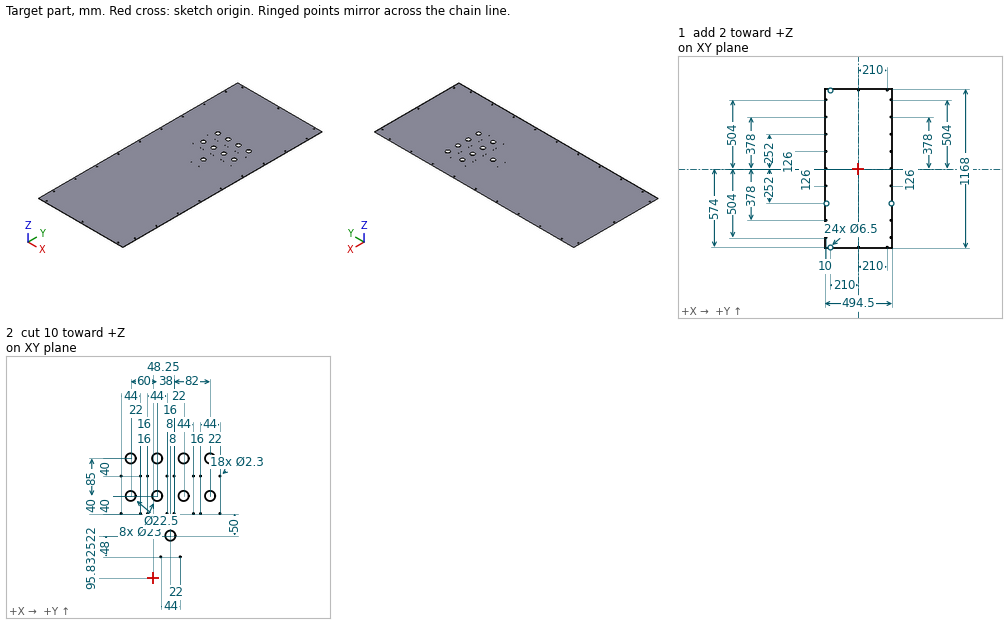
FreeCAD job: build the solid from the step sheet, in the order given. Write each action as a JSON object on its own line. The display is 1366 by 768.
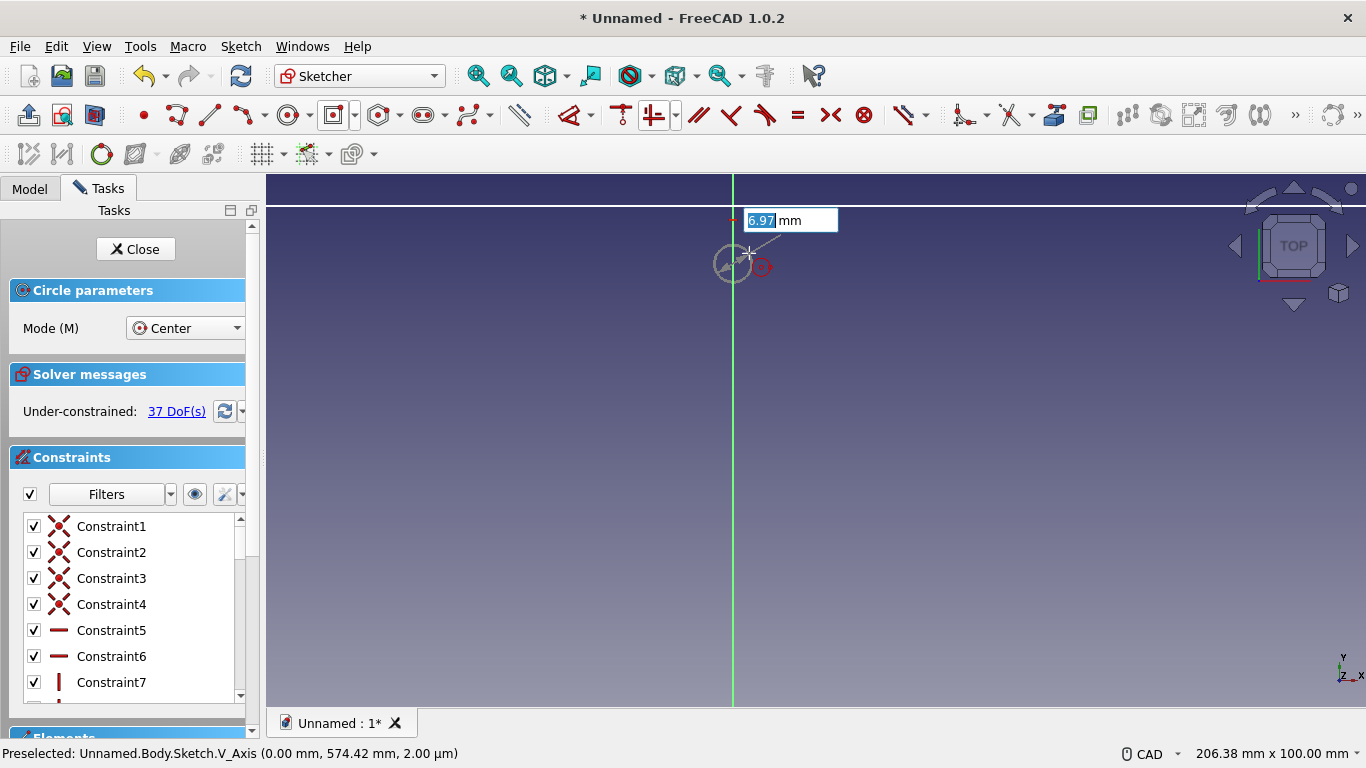
{"action": "type", "text": "6.5"}
{"action": "key", "text": "Return"}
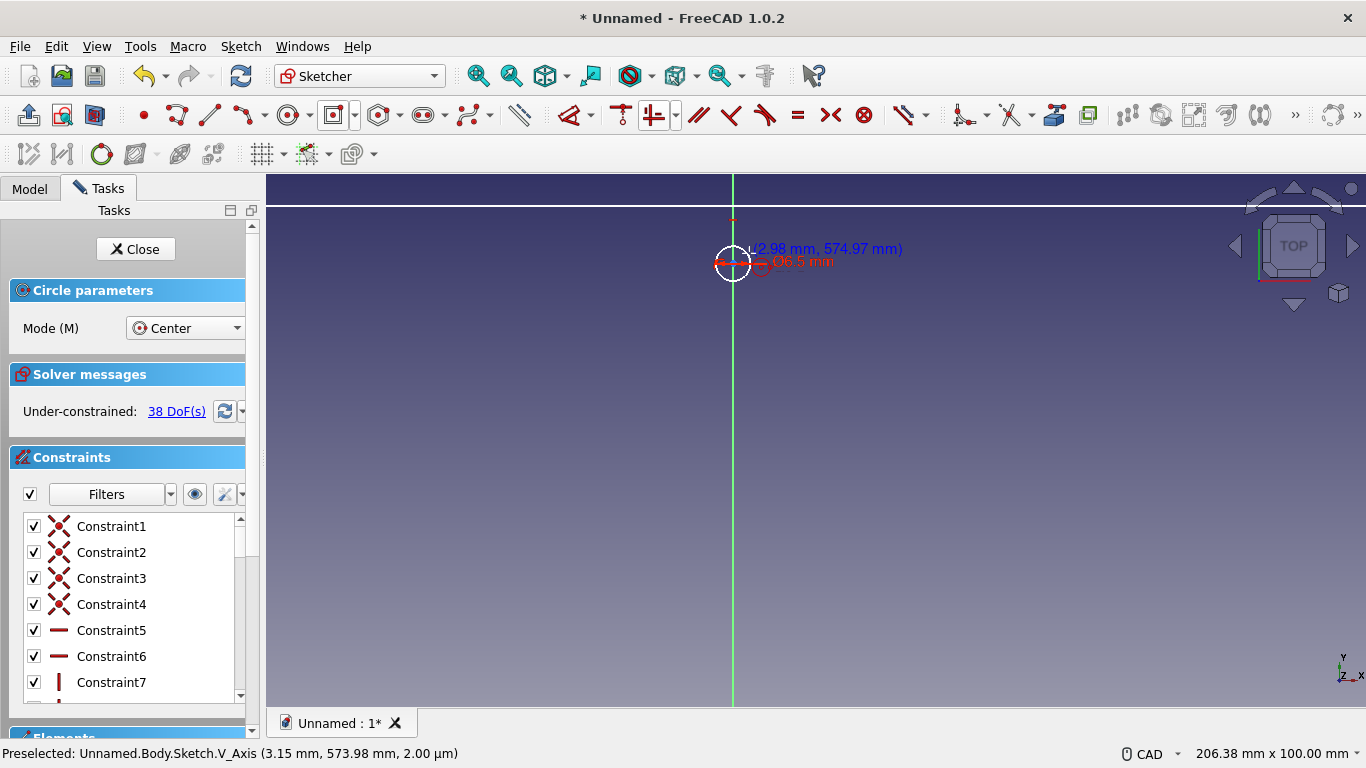
{"action": "scroll", "coordinate": [748, 290], "scroll_direction": "down", "scroll_amount": 15}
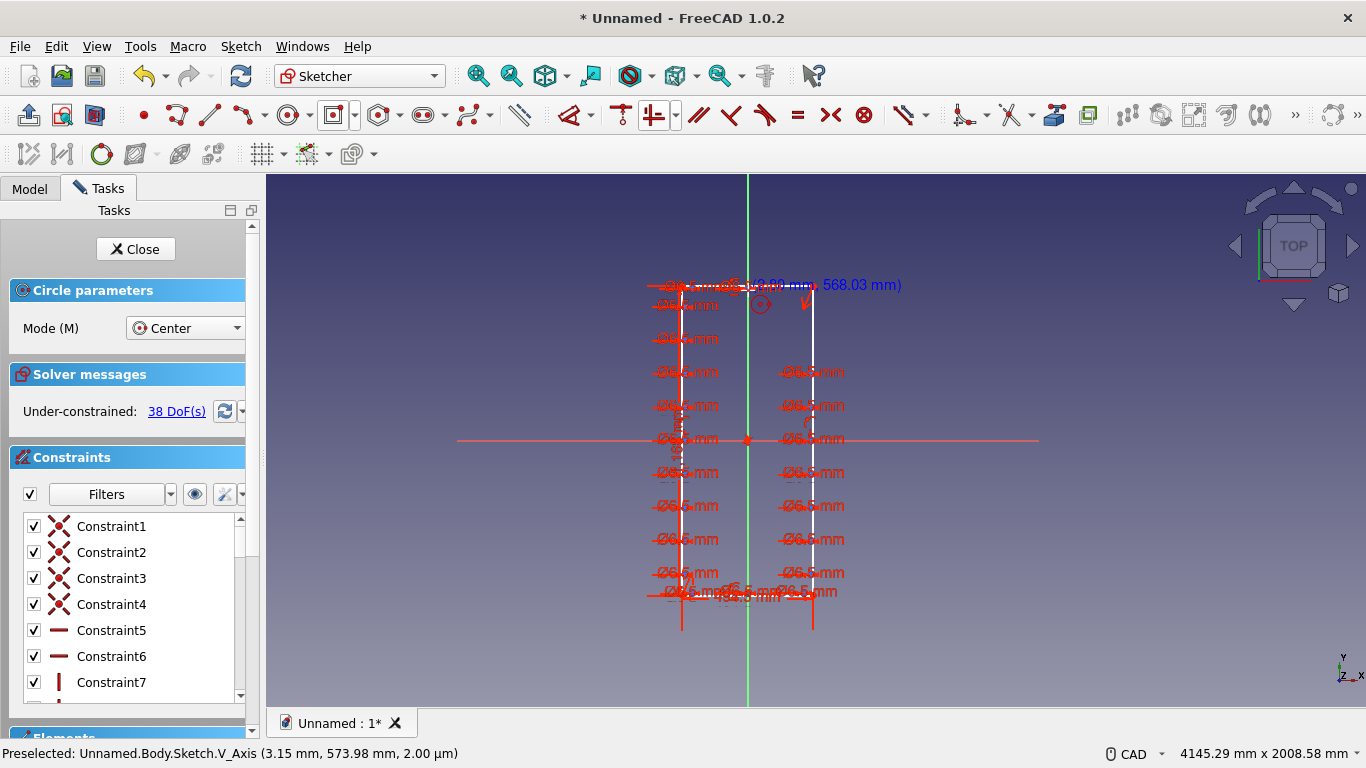
{"action": "scroll", "coordinate": [811, 341], "scroll_direction": "up", "scroll_amount": 17}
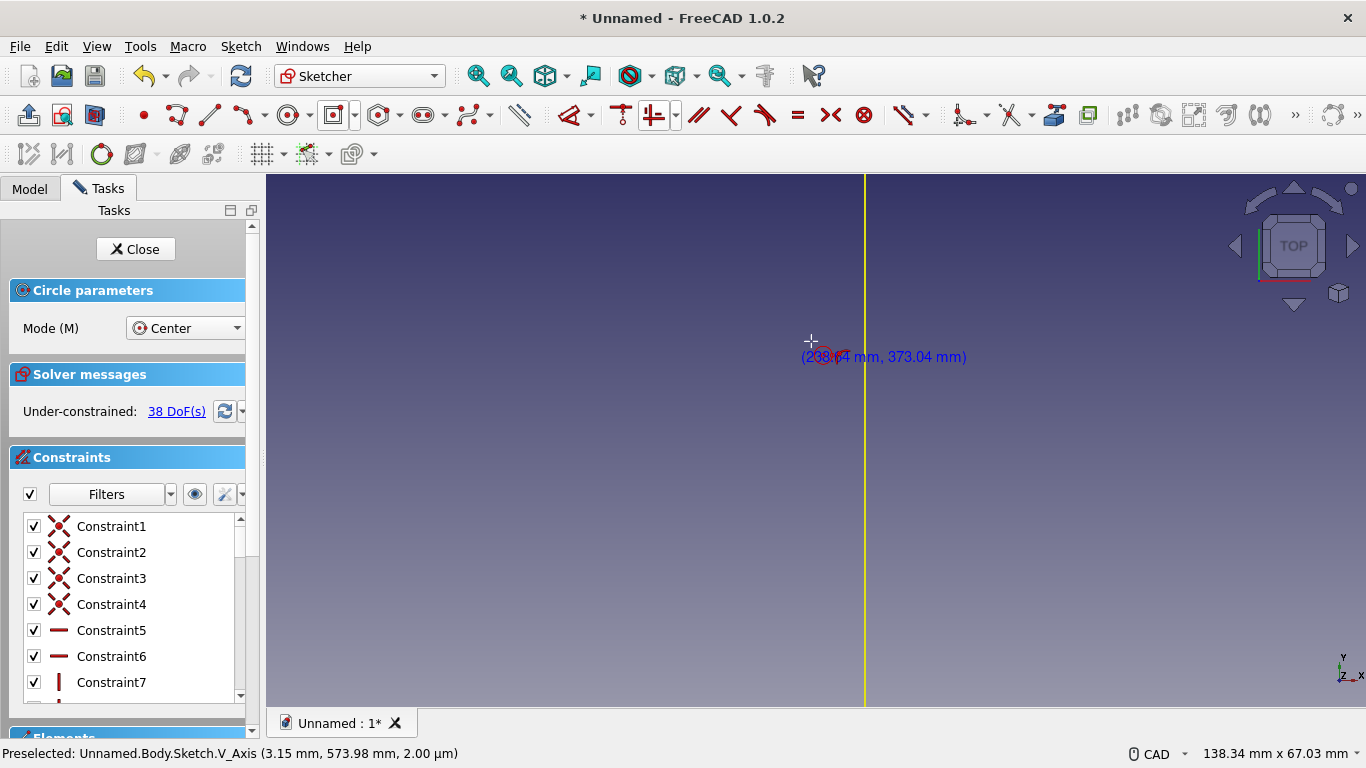
{"action": "scroll", "coordinate": [826, 318], "scroll_direction": "down", "scroll_amount": 16}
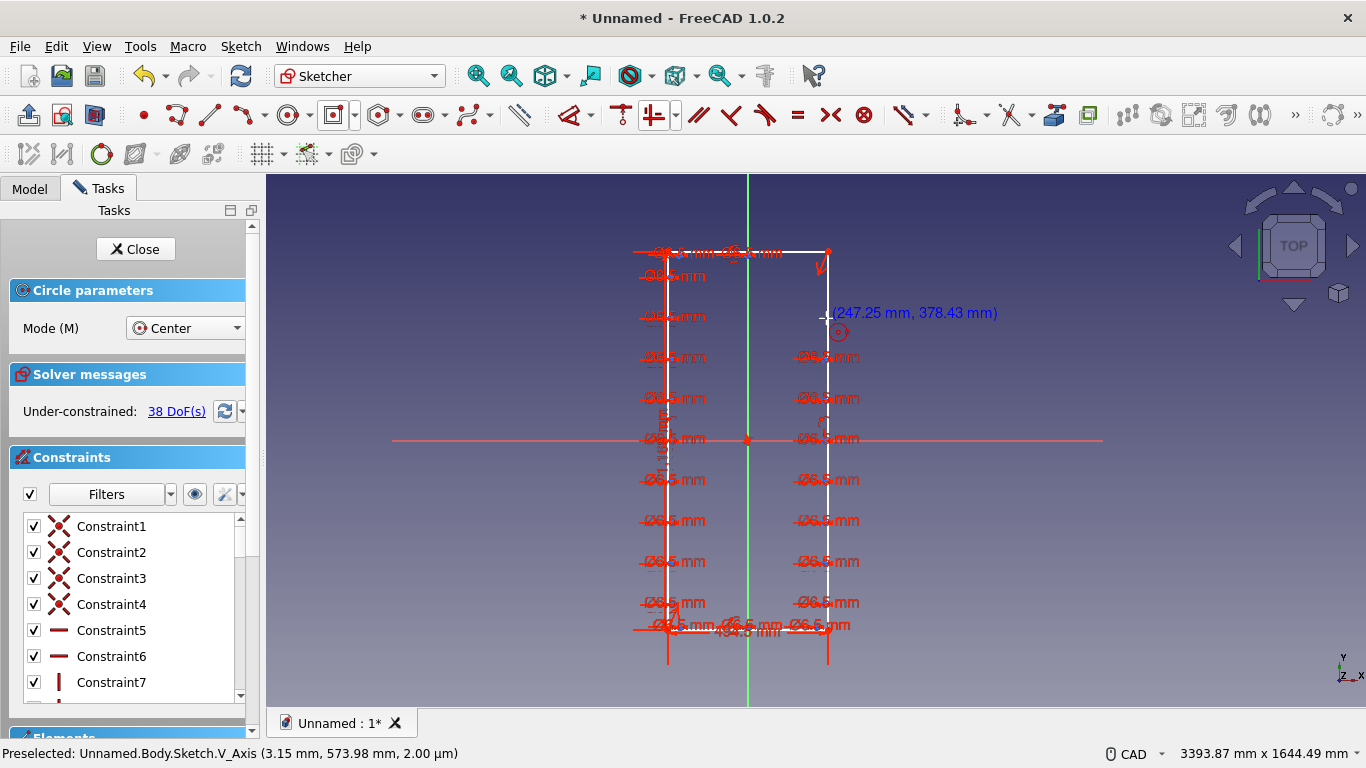
{"action": "scroll", "coordinate": [825, 318], "scroll_direction": "up", "scroll_amount": 8}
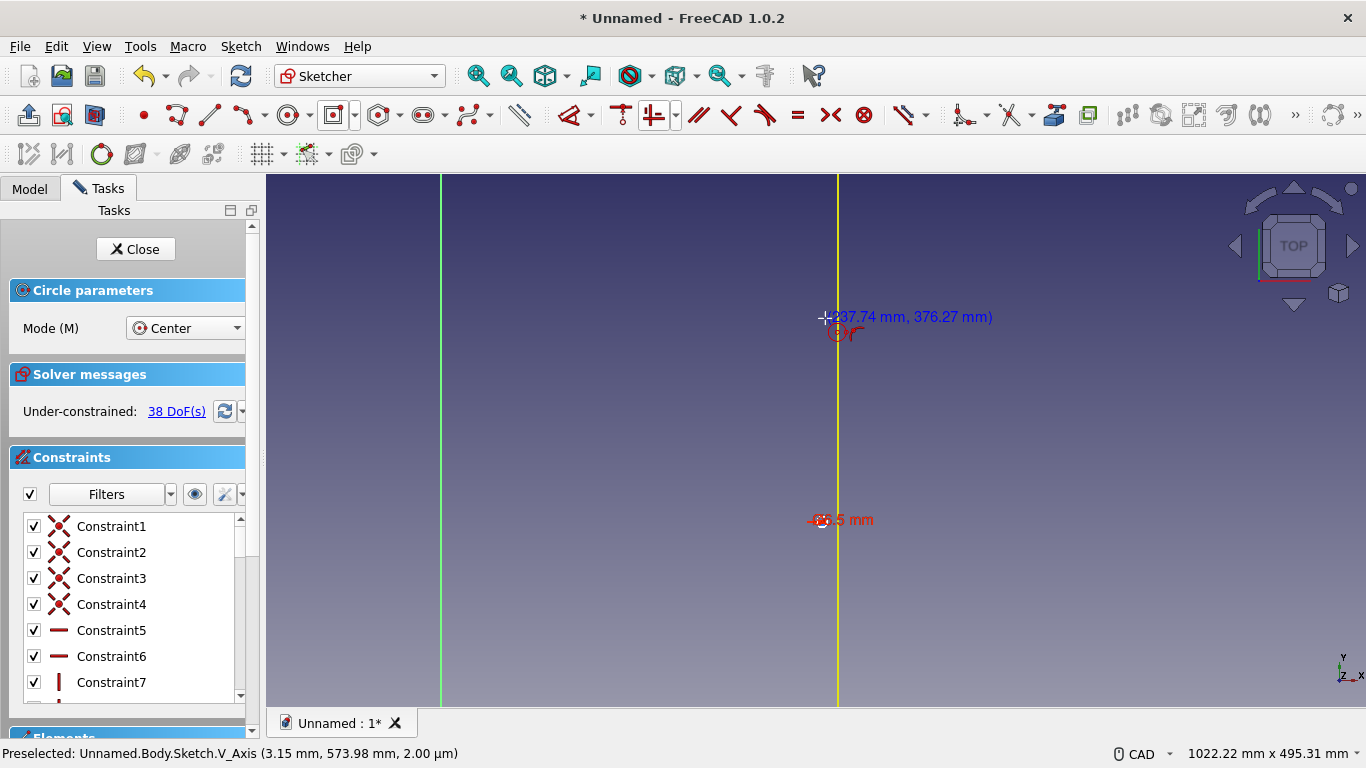
{"action": "left_click", "coordinate": [822, 319]}
{"action": "mouse_move", "coordinate": [819, 315]}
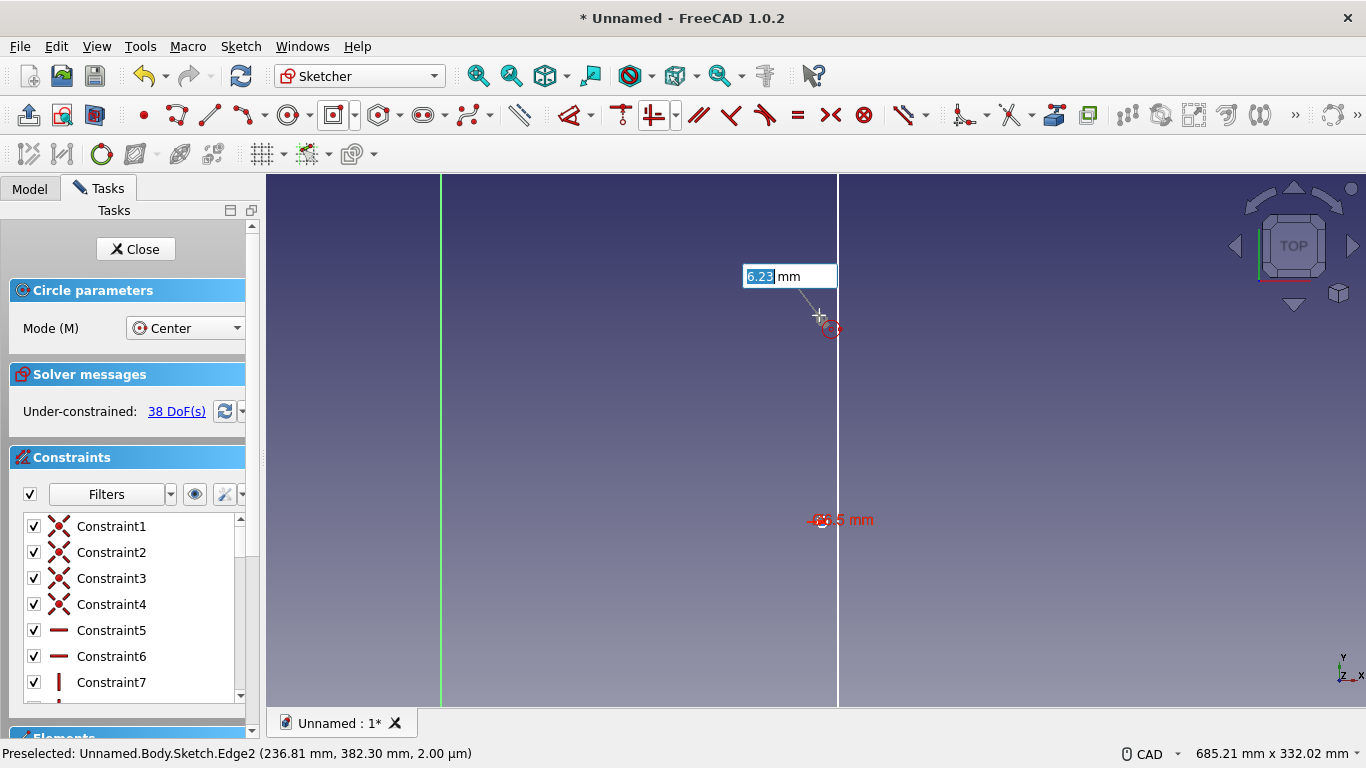
{"action": "type", "text": "6.5"}
{"action": "key", "text": "Return"}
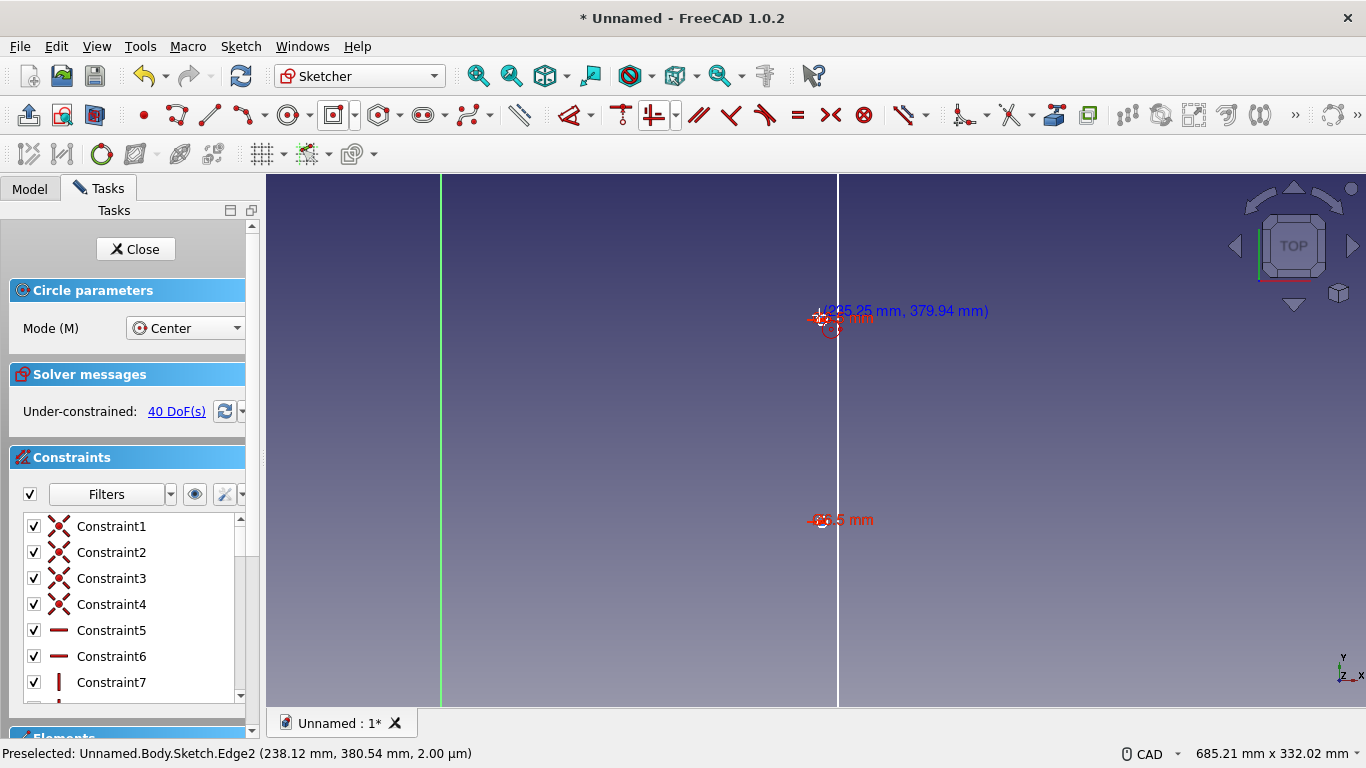
{"action": "scroll", "coordinate": [808, 344], "scroll_direction": "down", "scroll_amount": 9}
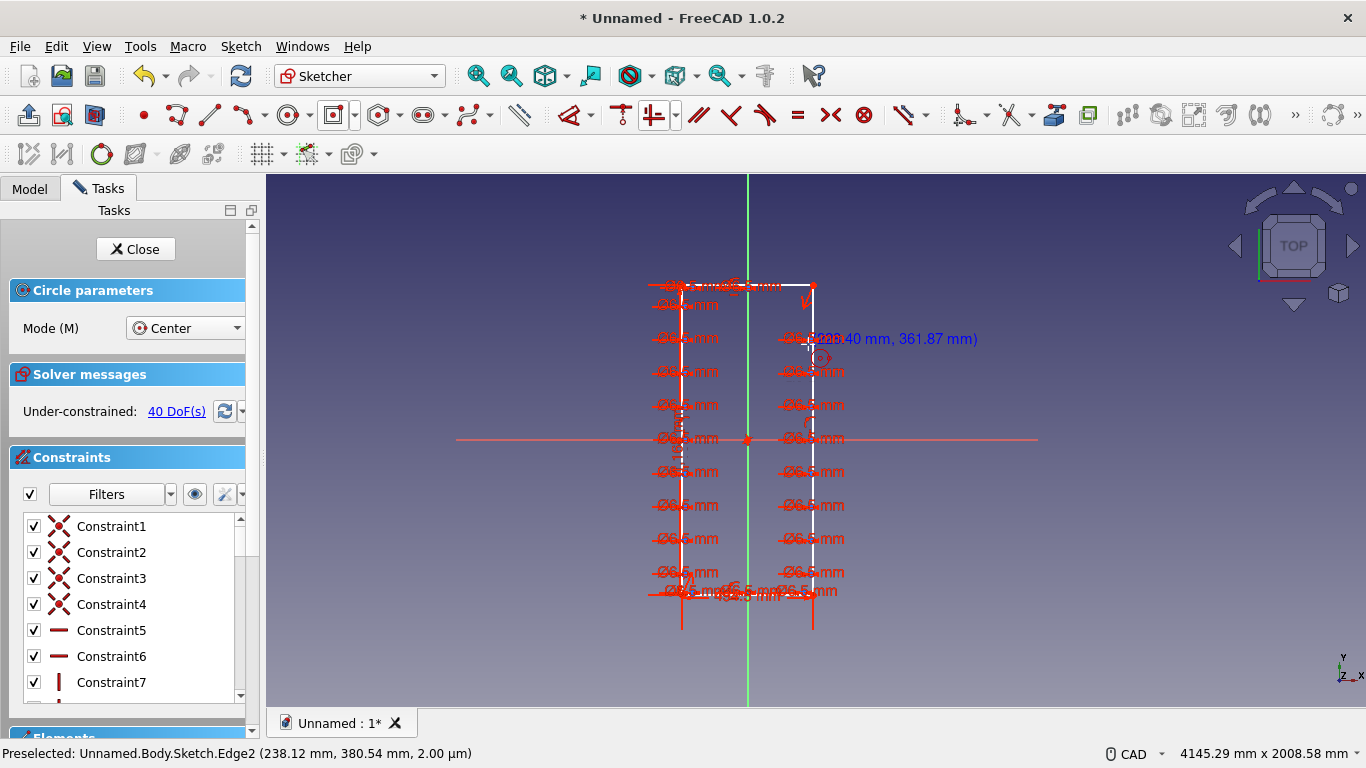
{"action": "scroll", "coordinate": [811, 307], "scroll_direction": "up", "scroll_amount": 17}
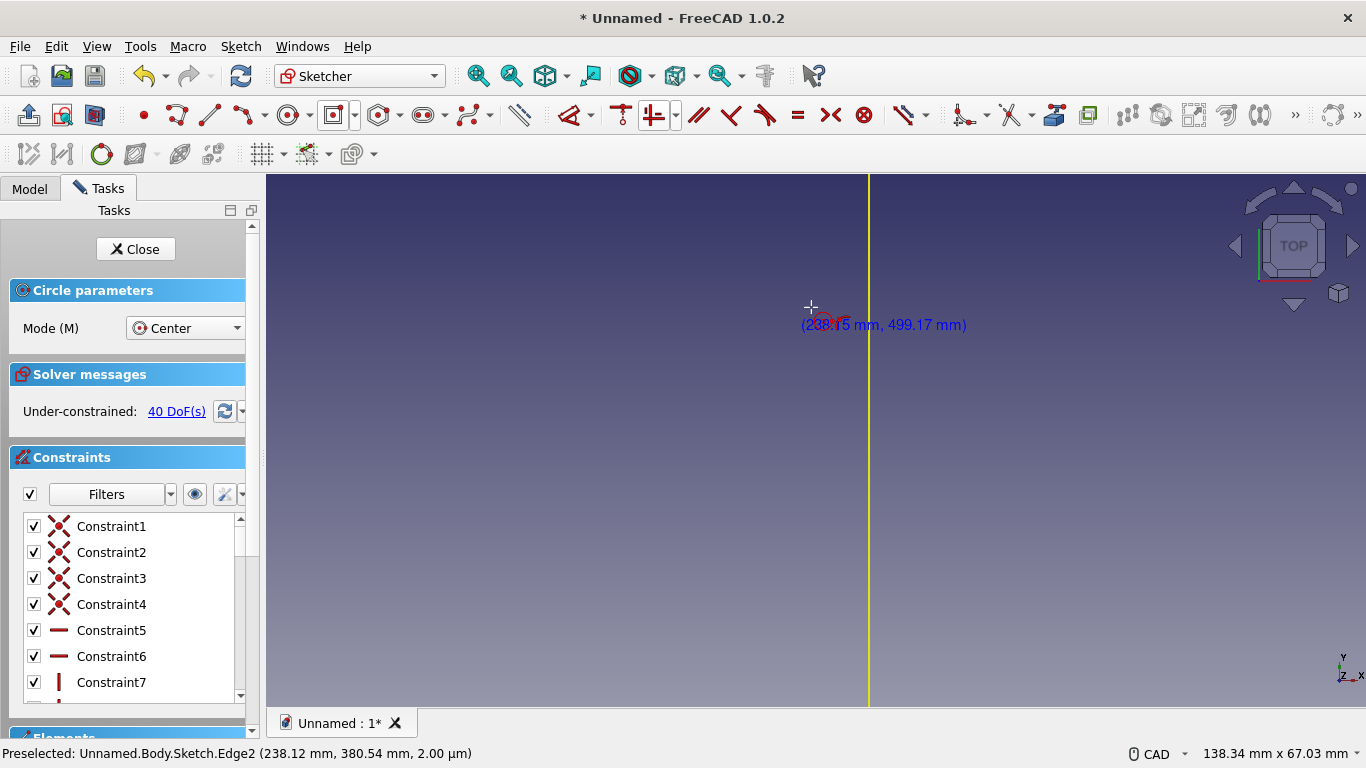
{"action": "scroll", "coordinate": [826, 277], "scroll_direction": "down", "scroll_amount": 16}